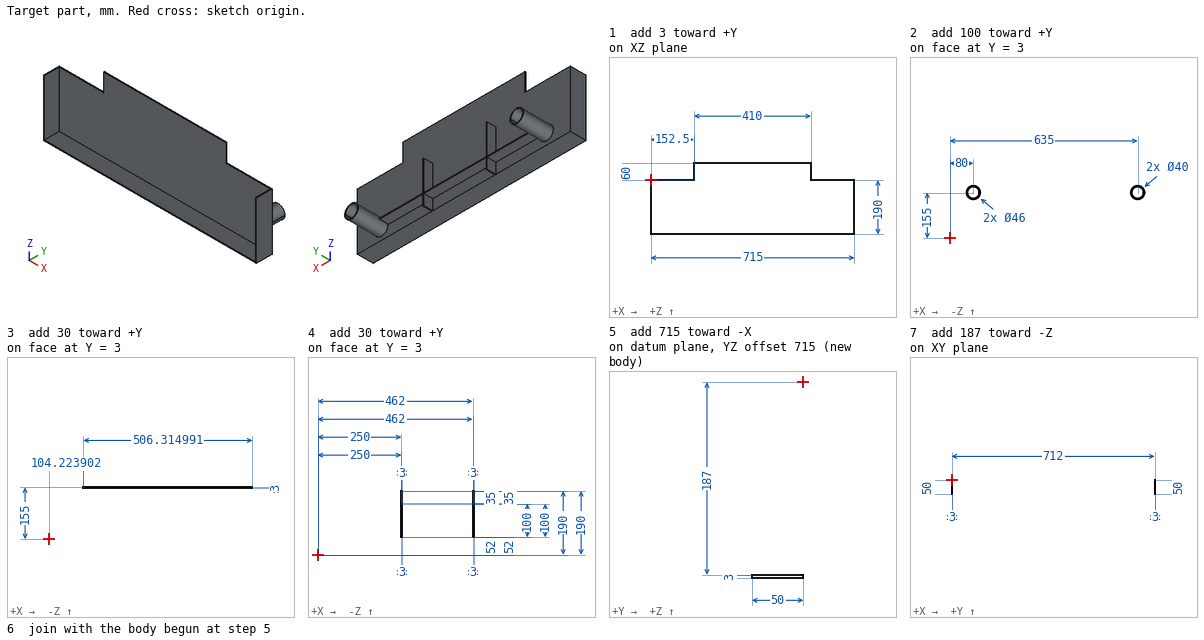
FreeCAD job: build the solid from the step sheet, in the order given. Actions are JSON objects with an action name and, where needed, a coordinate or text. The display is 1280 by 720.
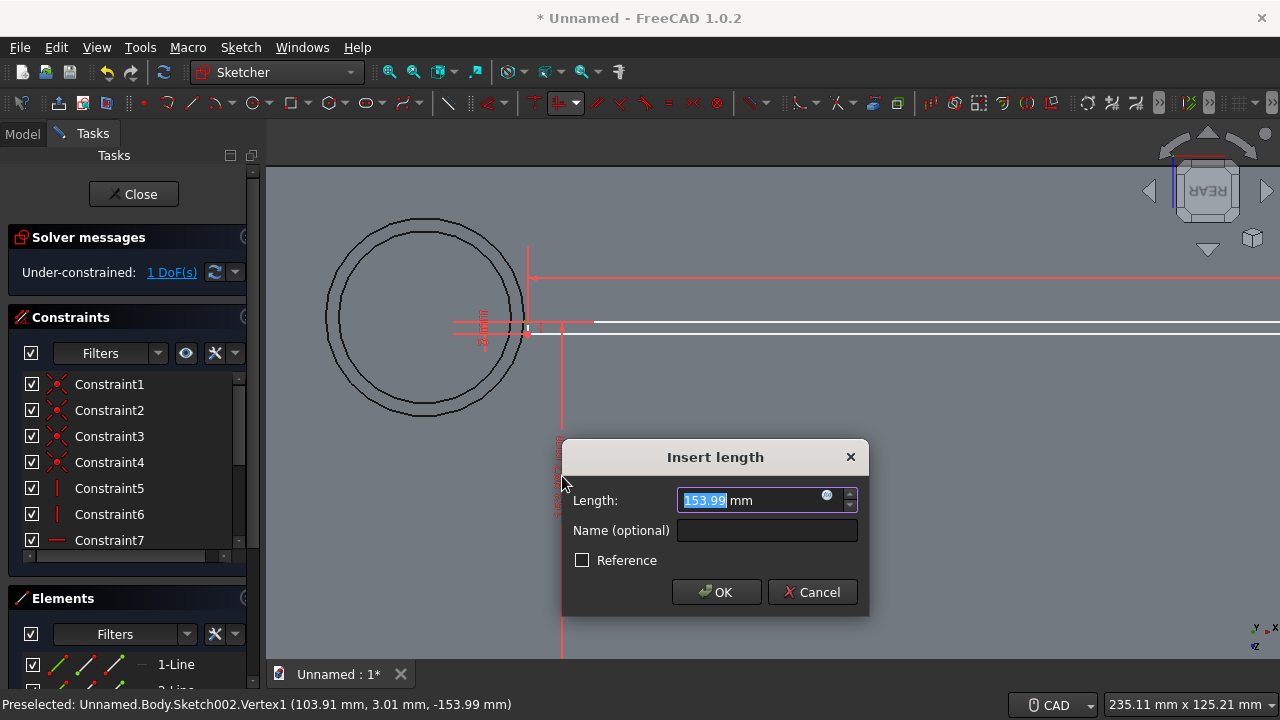
{"action": "type", "text": "155"}
{"action": "key", "text": "Return"}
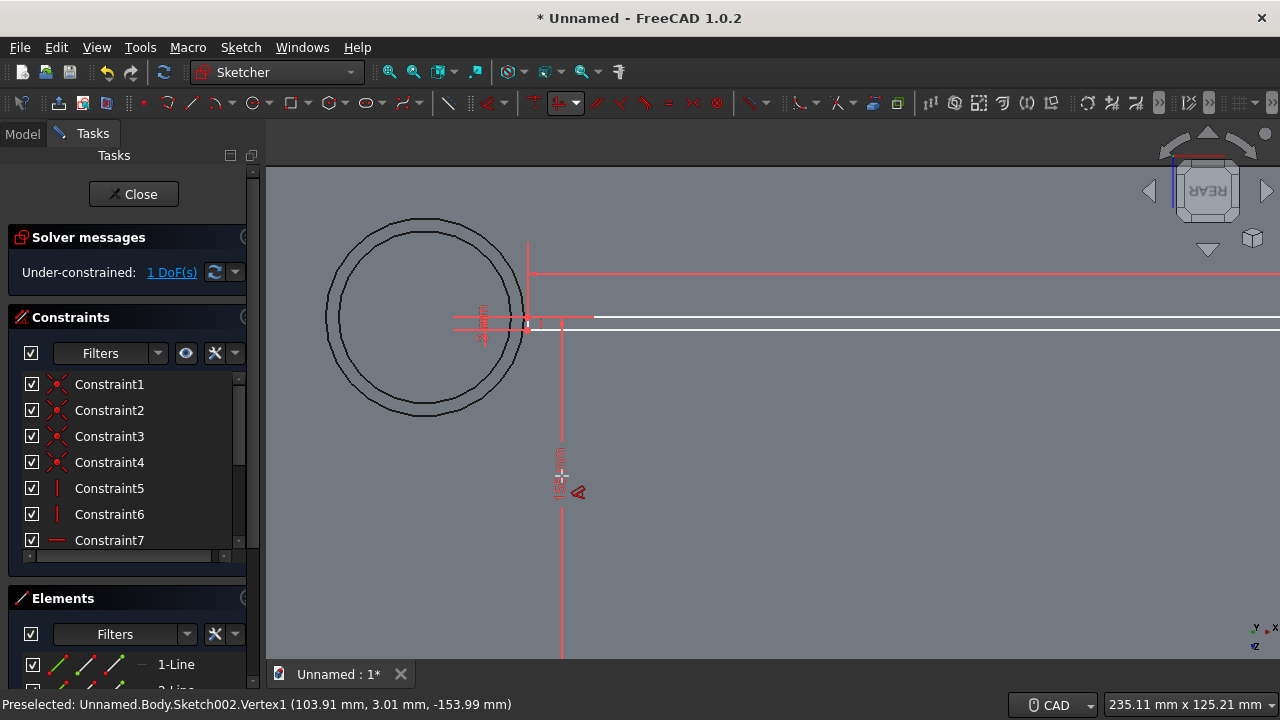
{"action": "left_click", "coordinate": [528, 317]}
{"action": "left_click", "coordinate": [411, 283]}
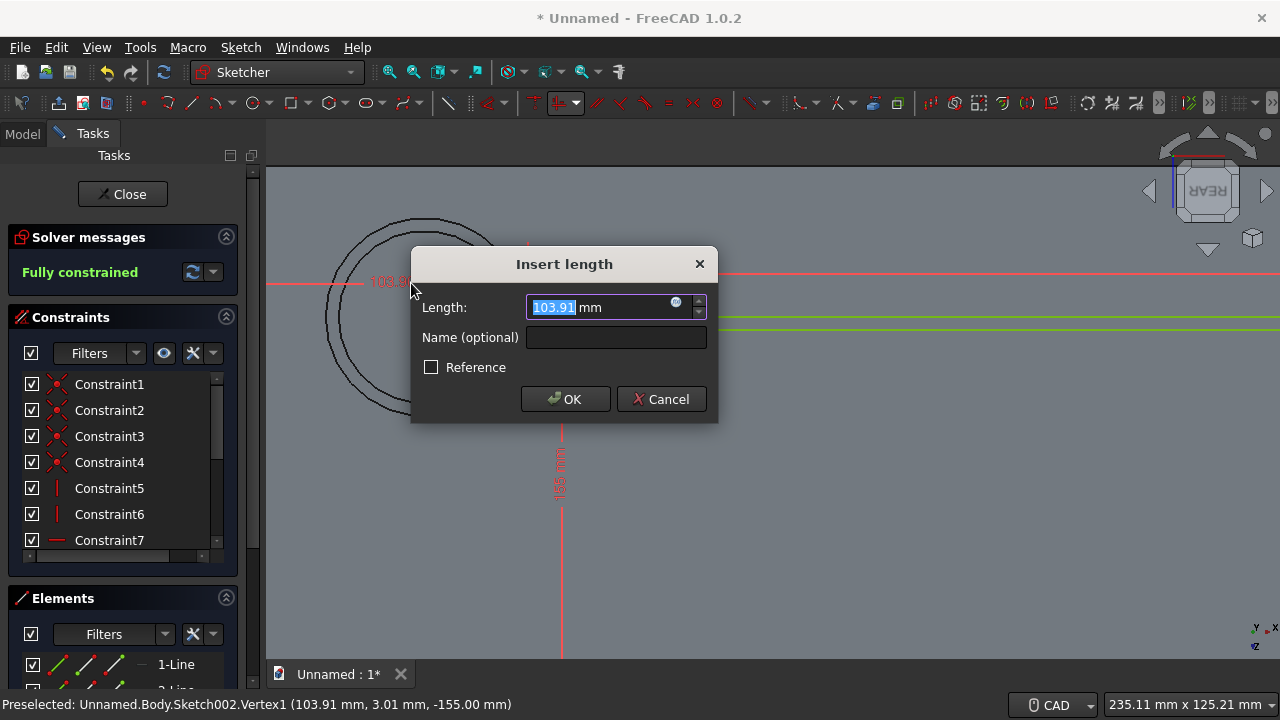
{"action": "type", "text": "104.223902"}
{"action": "key", "text": "Return"}
{"action": "key", "text": "Escape"}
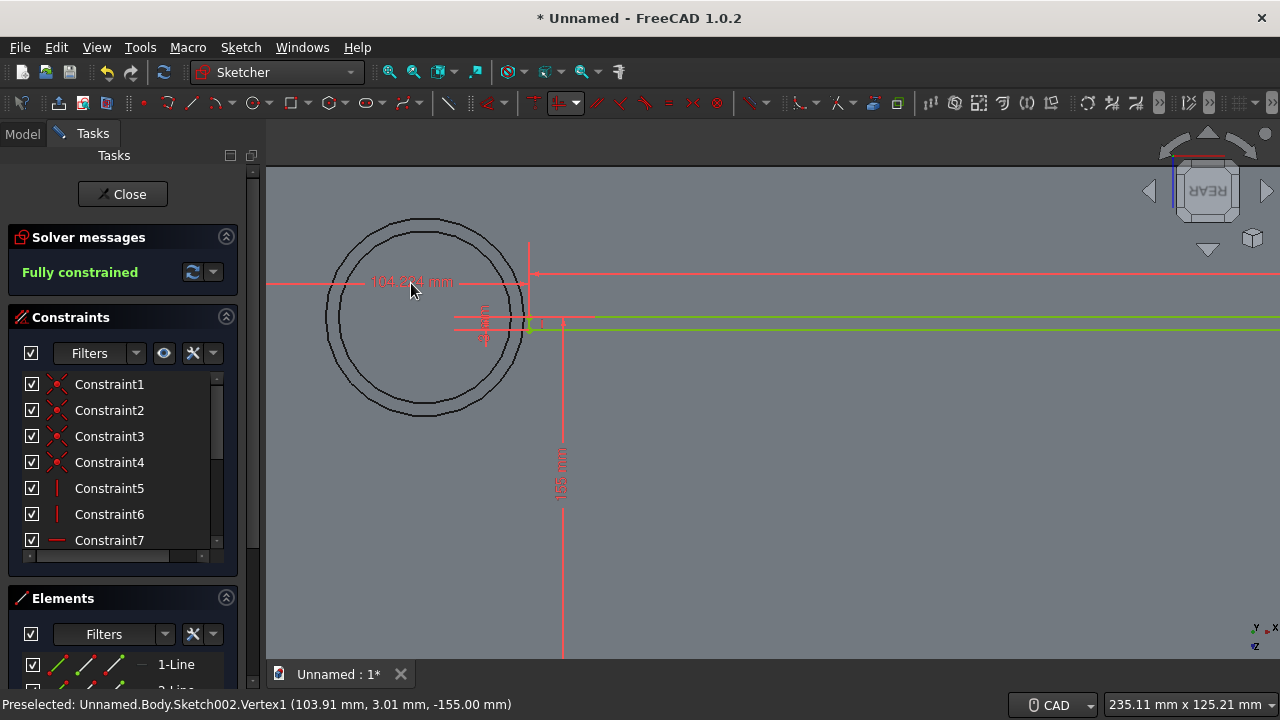
{"action": "left_click", "coordinate": [123, 194]}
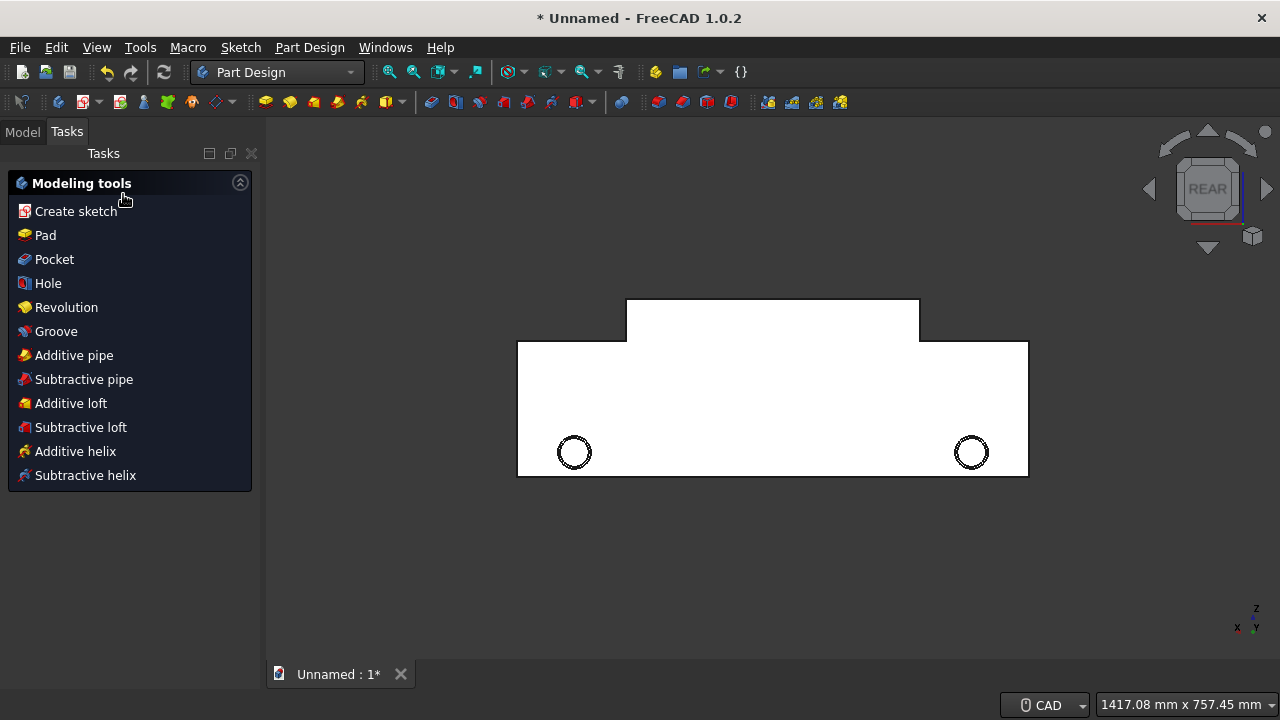
{"action": "left_click", "coordinate": [266, 102]}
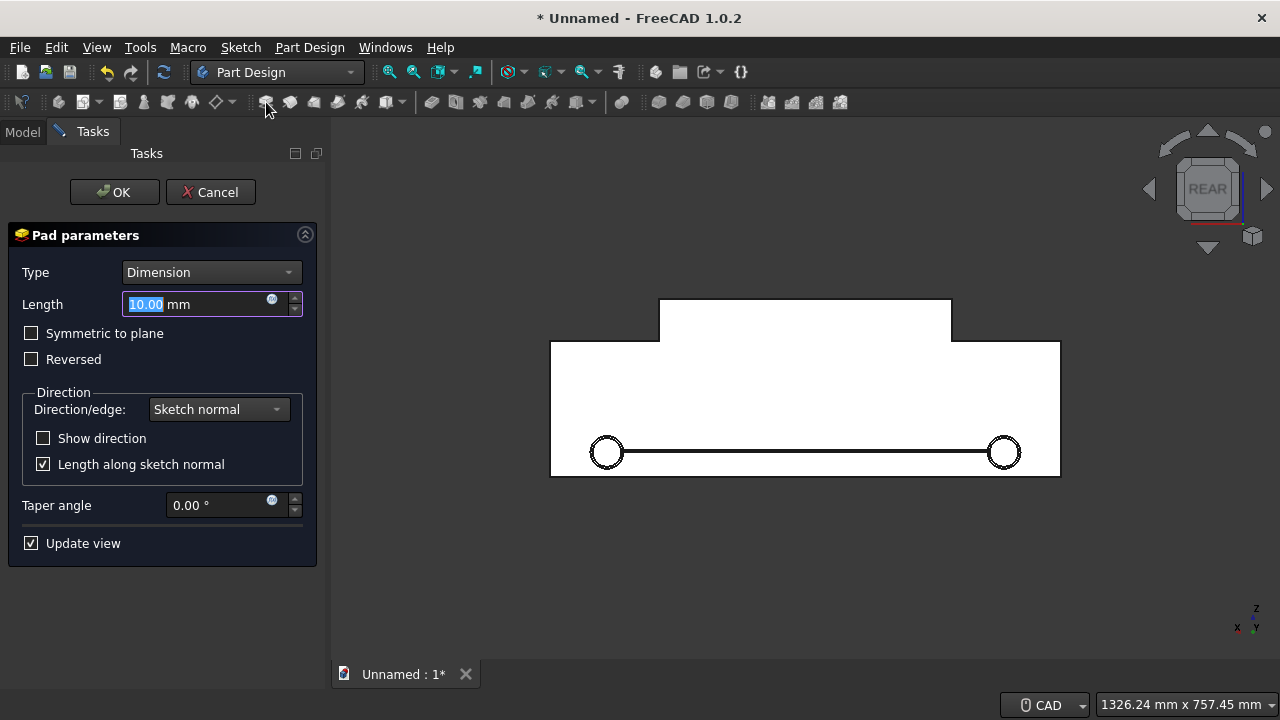
{"action": "type", "text": "30"}
{"action": "key", "text": "Tab"}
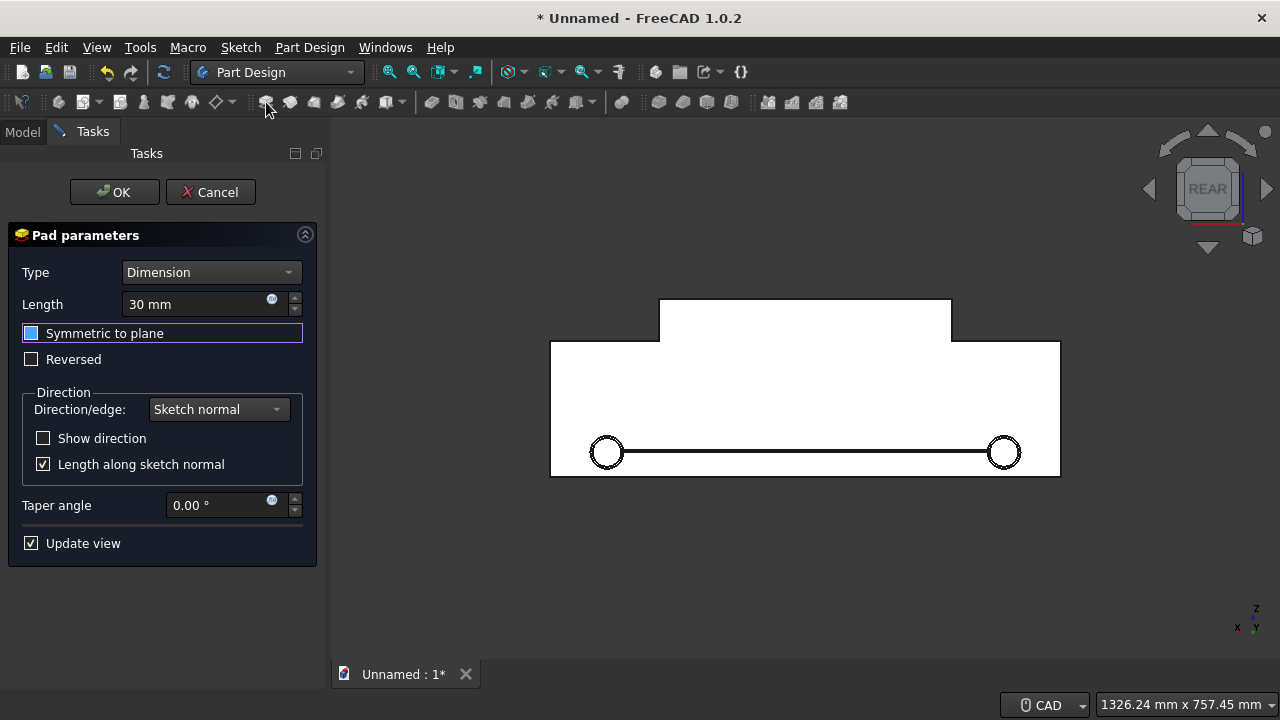
{"action": "left_click", "coordinate": [115, 192]}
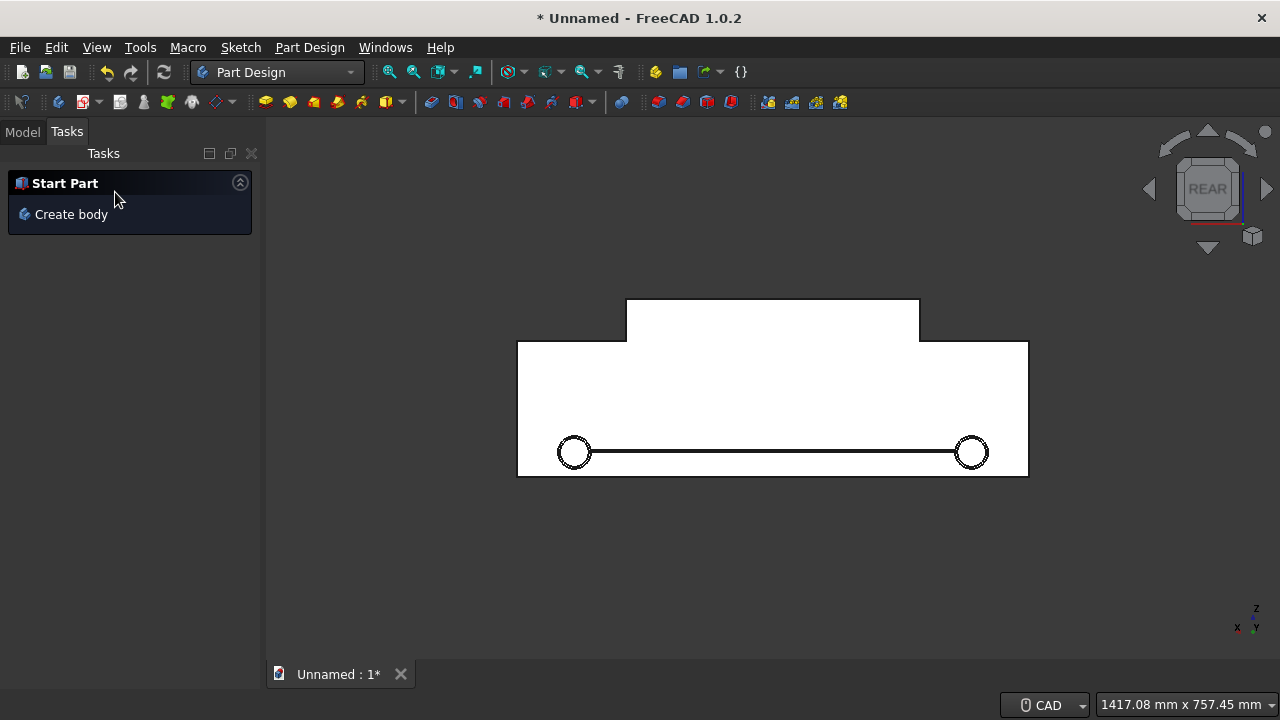
{"action": "left_click", "coordinate": [700, 361]}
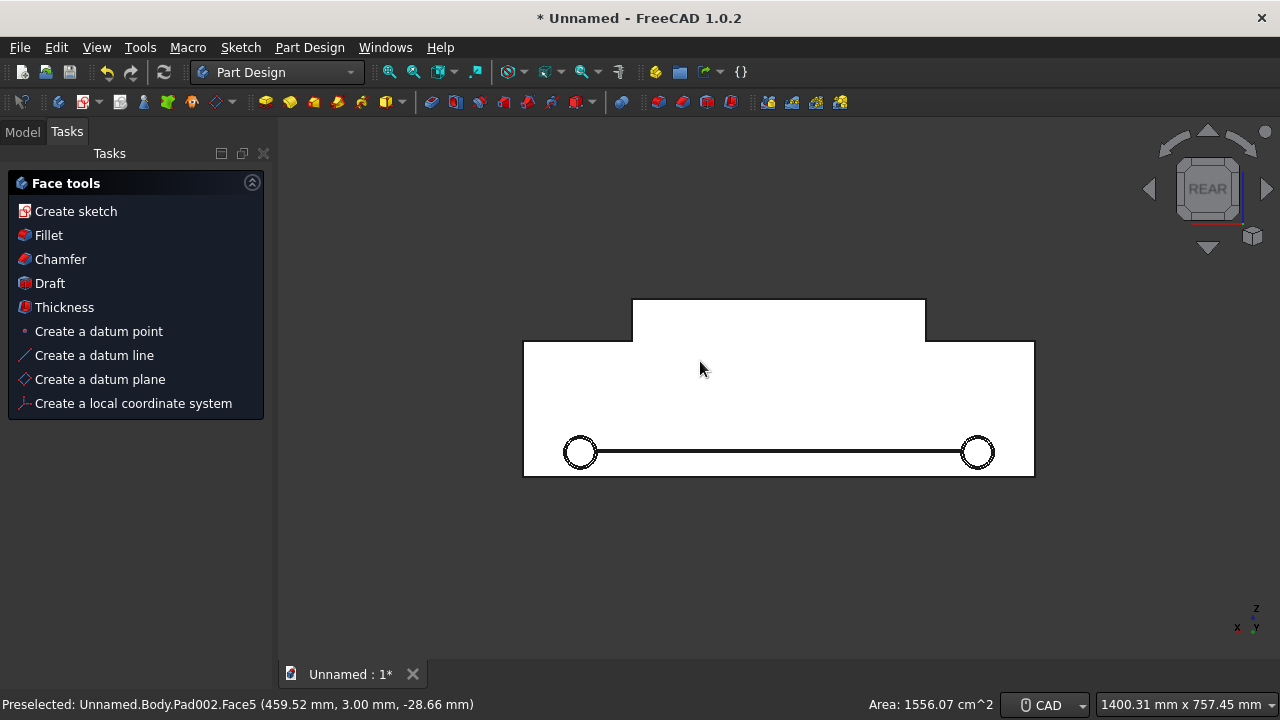
{"action": "left_click", "coordinate": [84, 102]}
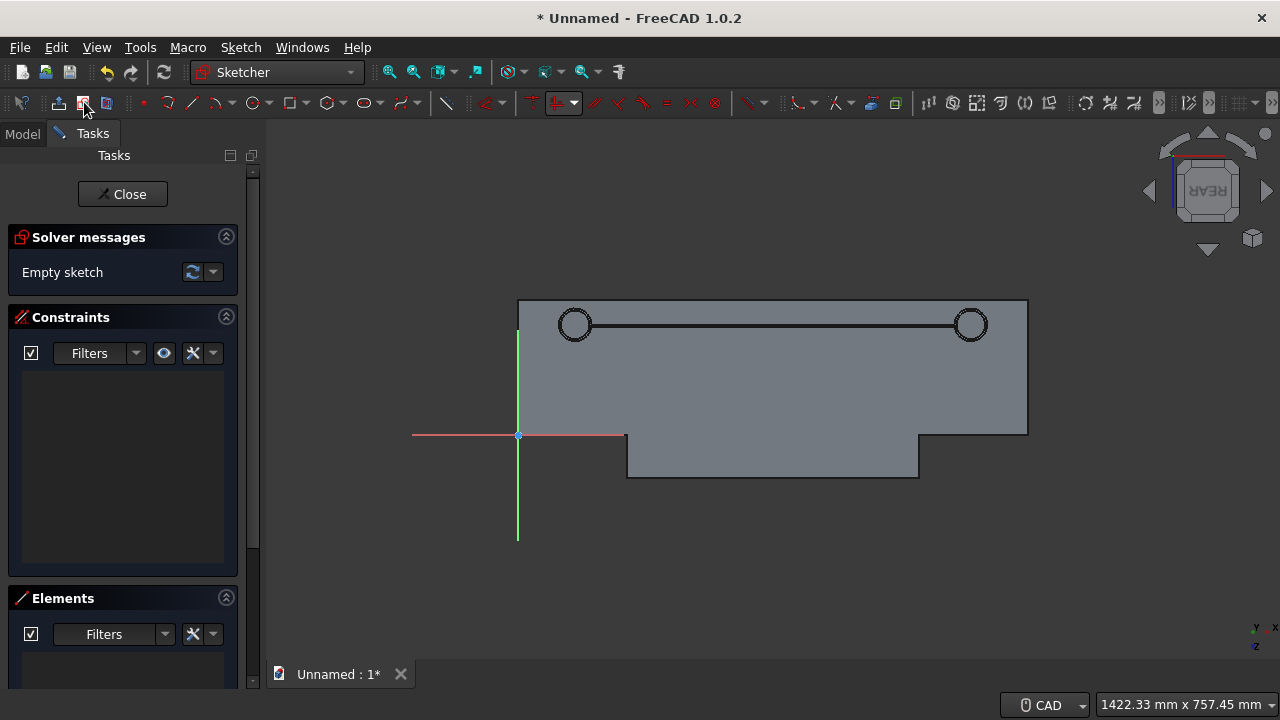
{"action": "scroll", "coordinate": [659, 342], "scroll_direction": "up", "scroll_amount": 3}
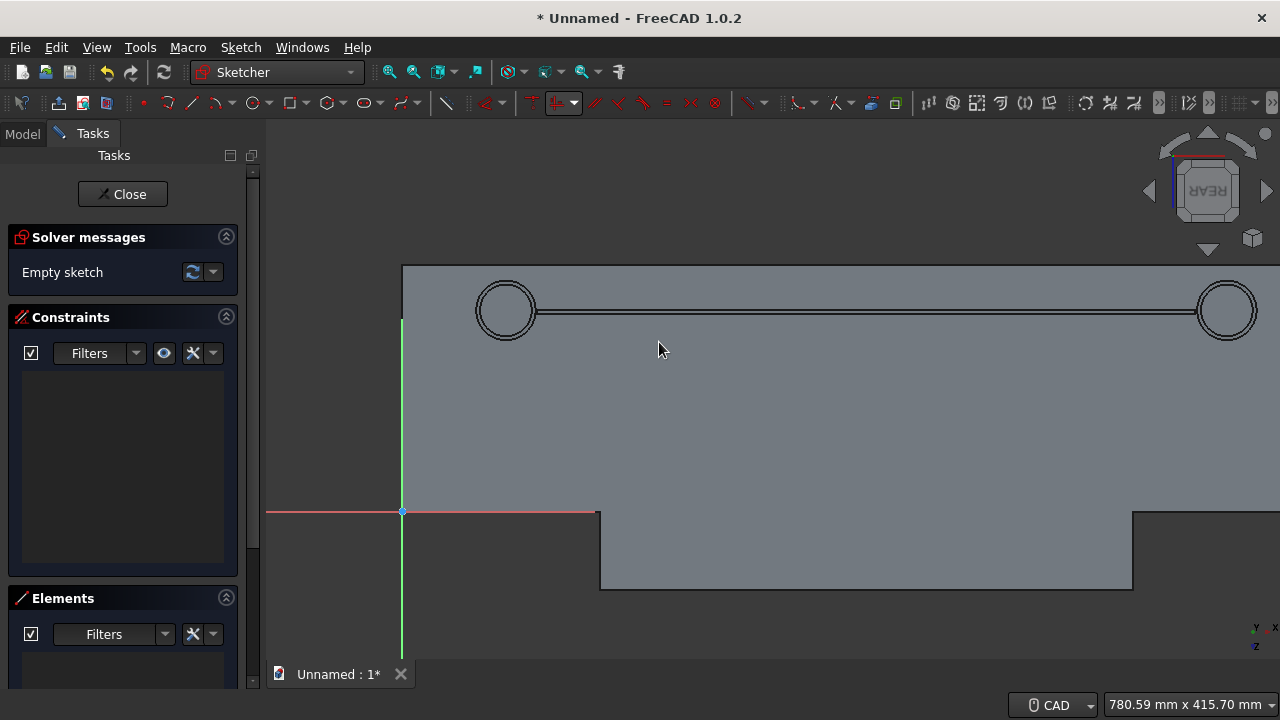
{"action": "key", "text": "g r"}